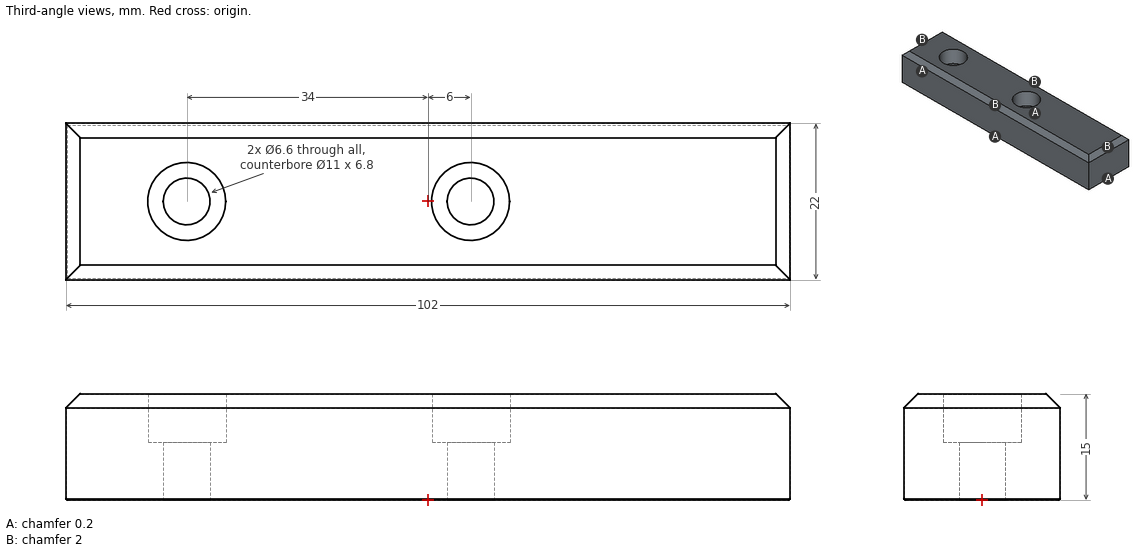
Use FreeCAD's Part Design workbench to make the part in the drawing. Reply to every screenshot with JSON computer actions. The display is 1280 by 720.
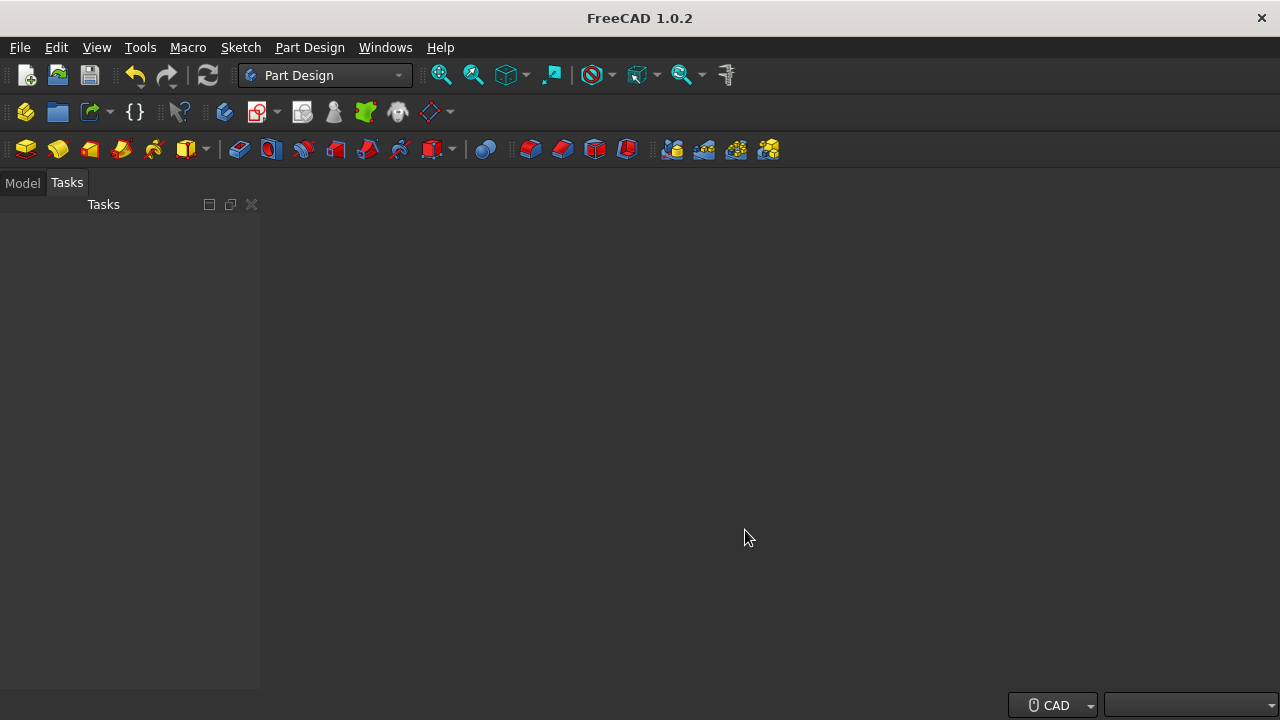
{"action": "left_click", "coordinate": [26, 76]}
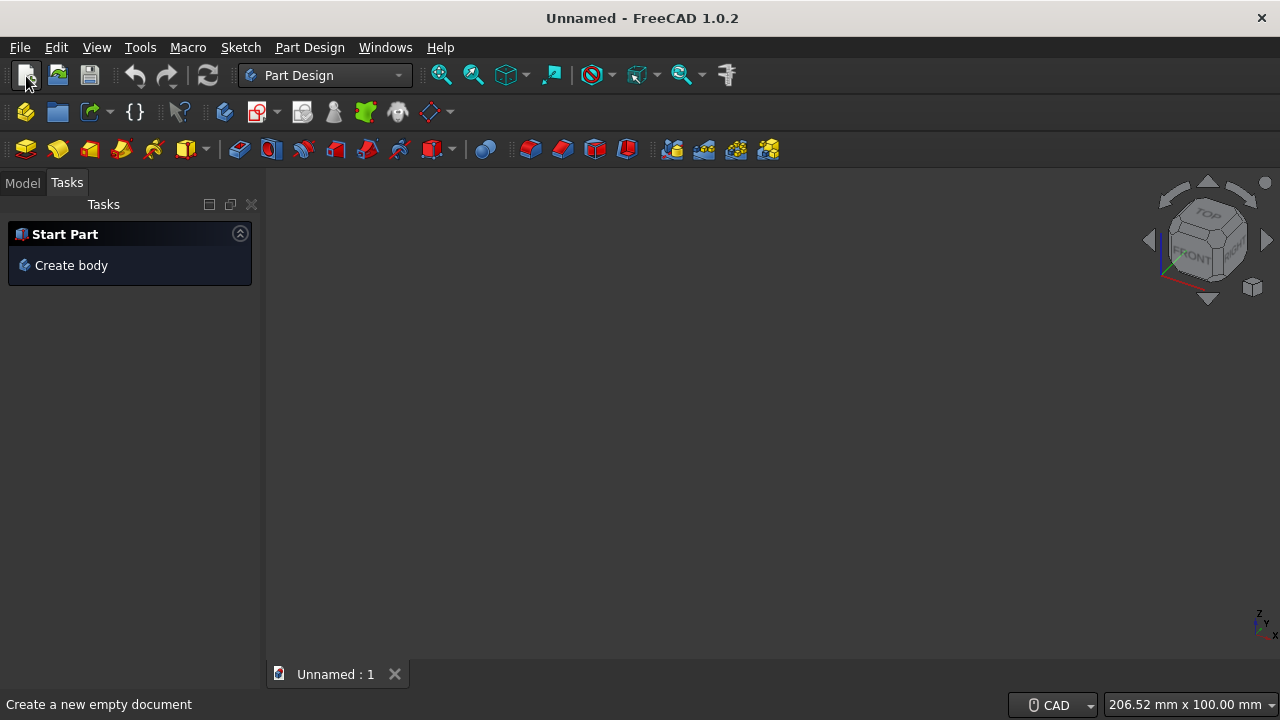
{"action": "left_click", "coordinate": [258, 112]}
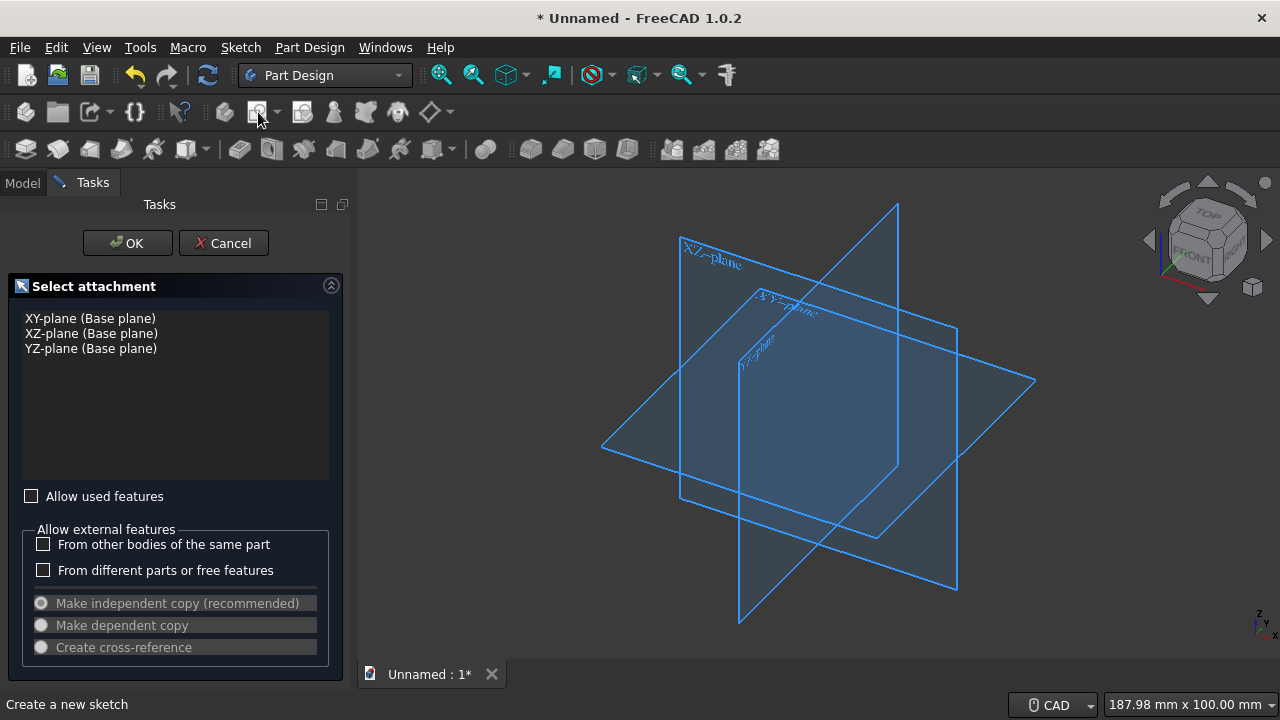
{"action": "left_click", "coordinate": [82, 318]}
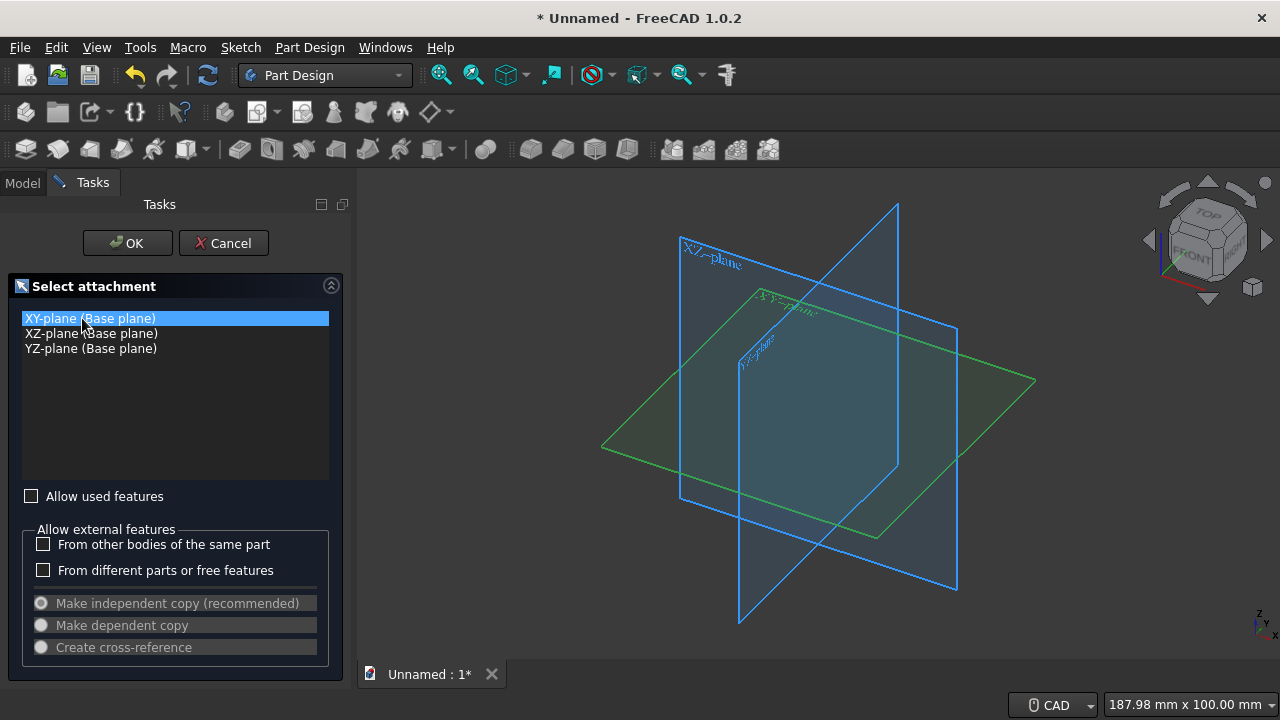
{"action": "left_click", "coordinate": [128, 243]}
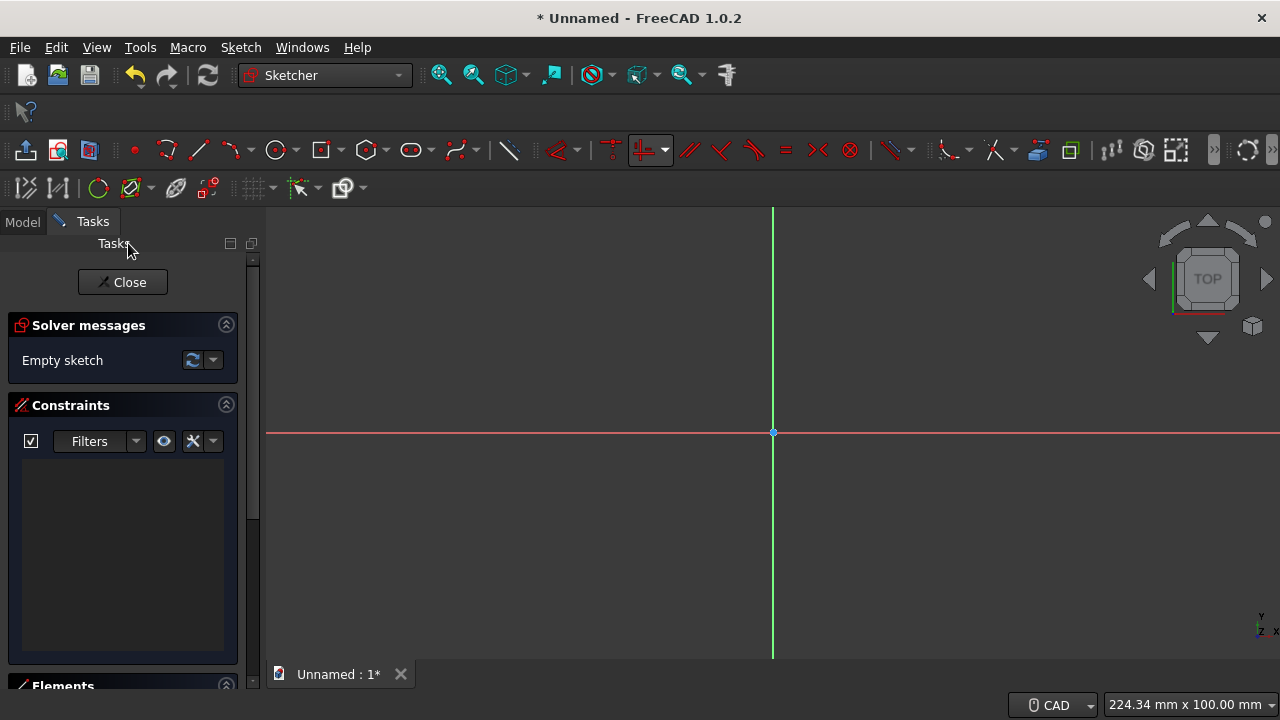
{"action": "left_click", "coordinate": [322, 150]}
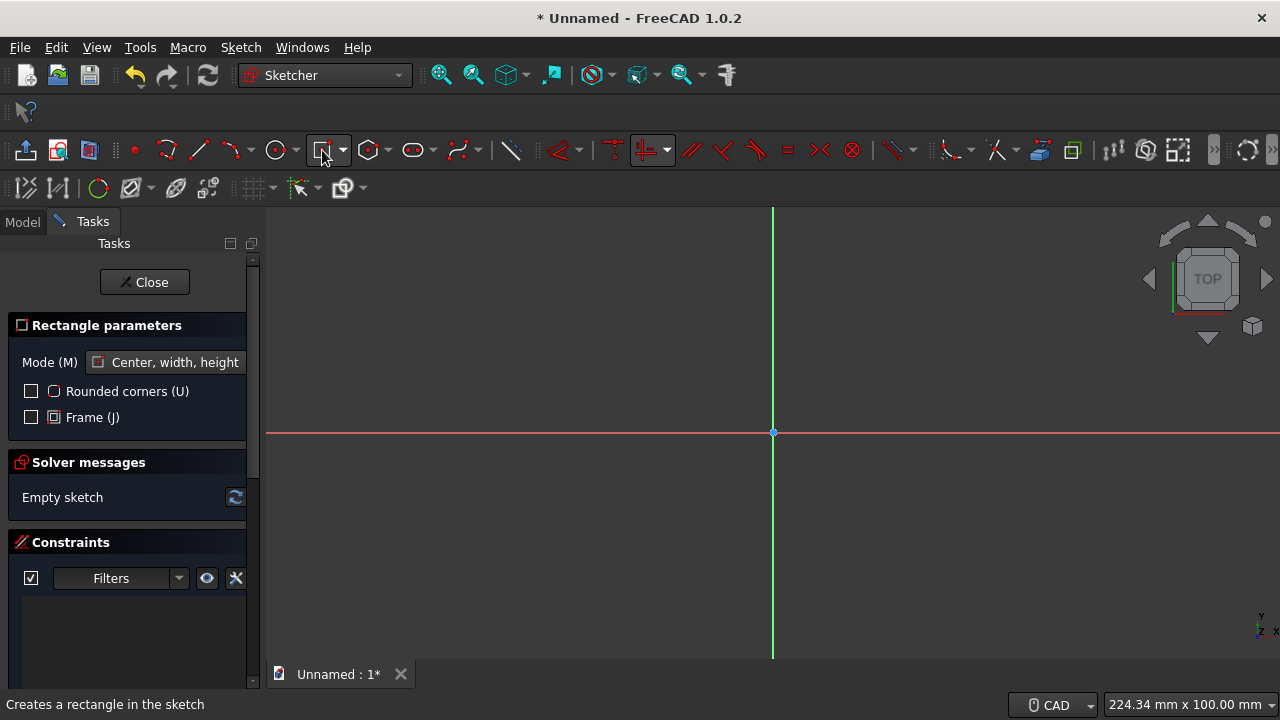
{"action": "left_click", "coordinate": [773, 433]}
{"action": "mouse_move", "coordinate": [1004, 383]}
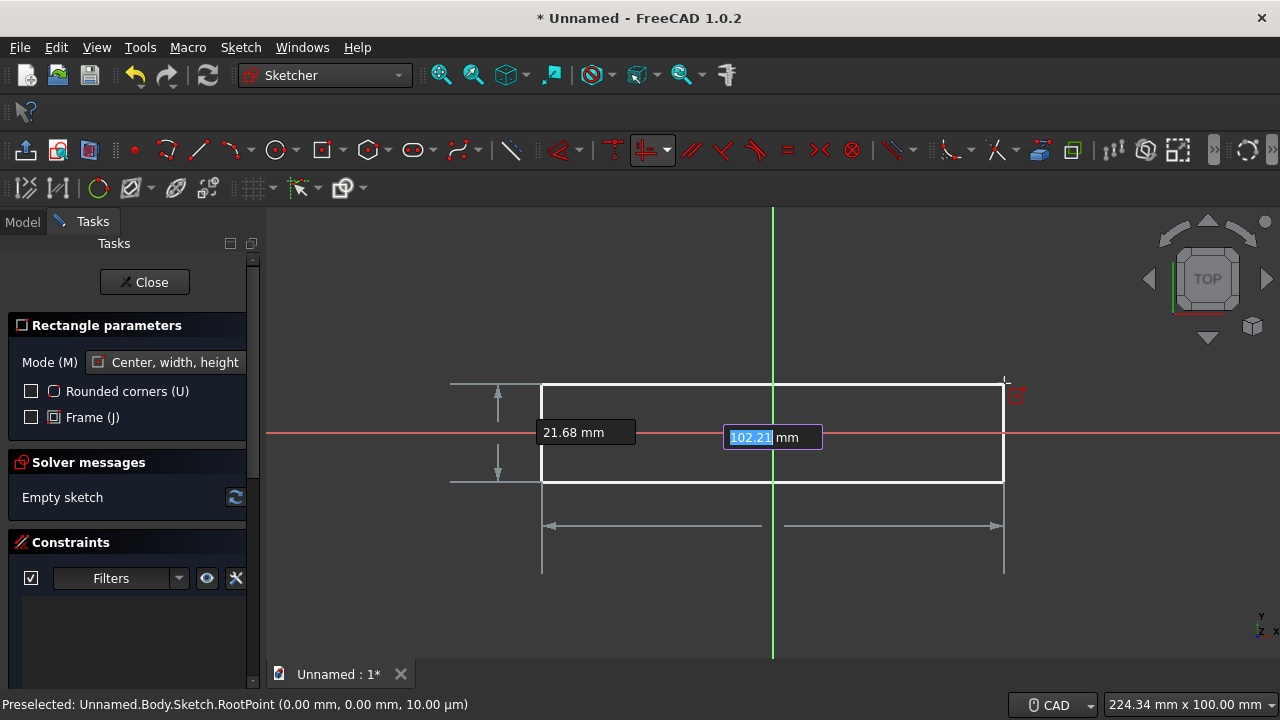
{"action": "type", "text": "102"}
{"action": "key", "text": "Tab"}
{"action": "type", "text": "22"}
{"action": "key", "text": "Return"}
{"action": "key", "text": "Escape"}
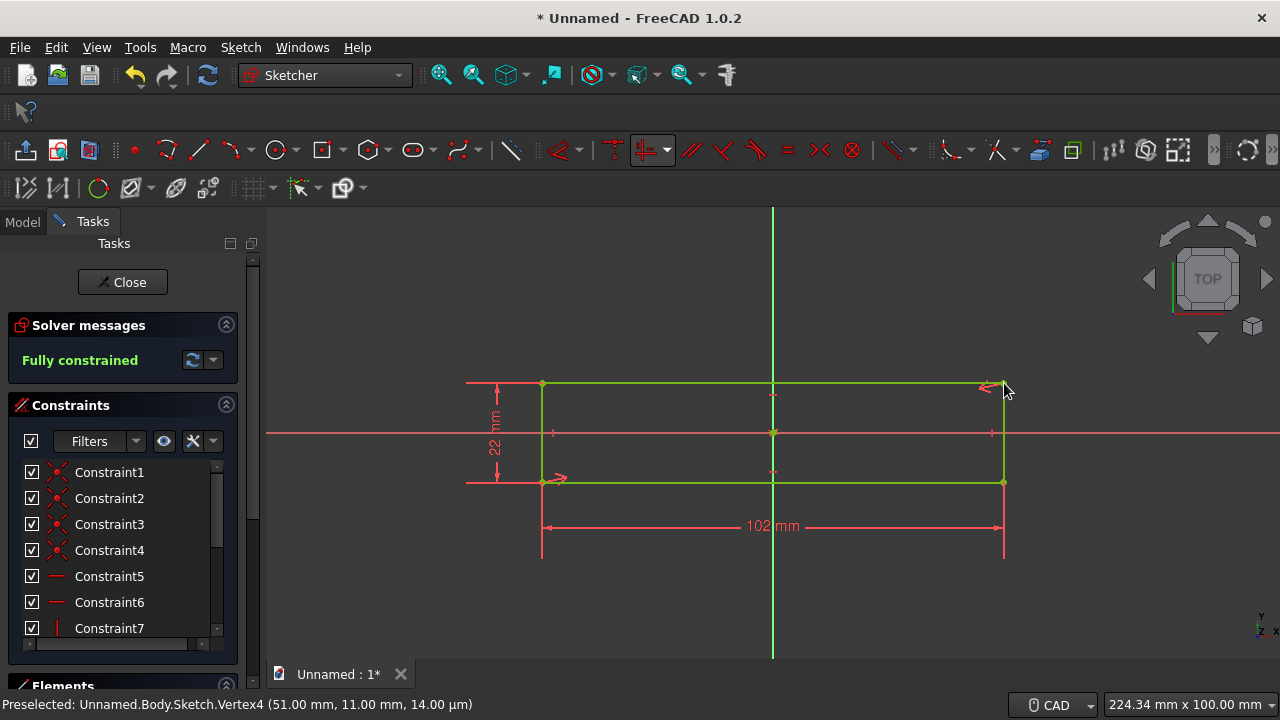
{"action": "left_click", "coordinate": [123, 282]}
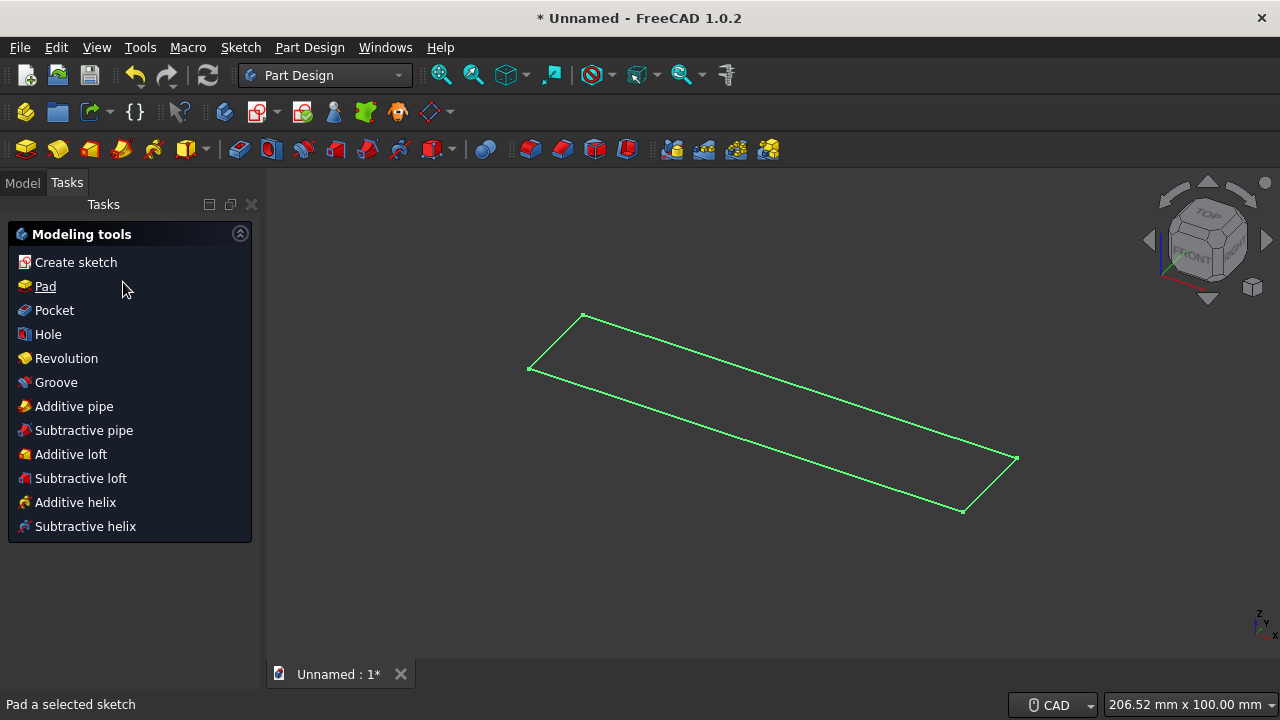
{"action": "left_click", "coordinate": [26, 150]}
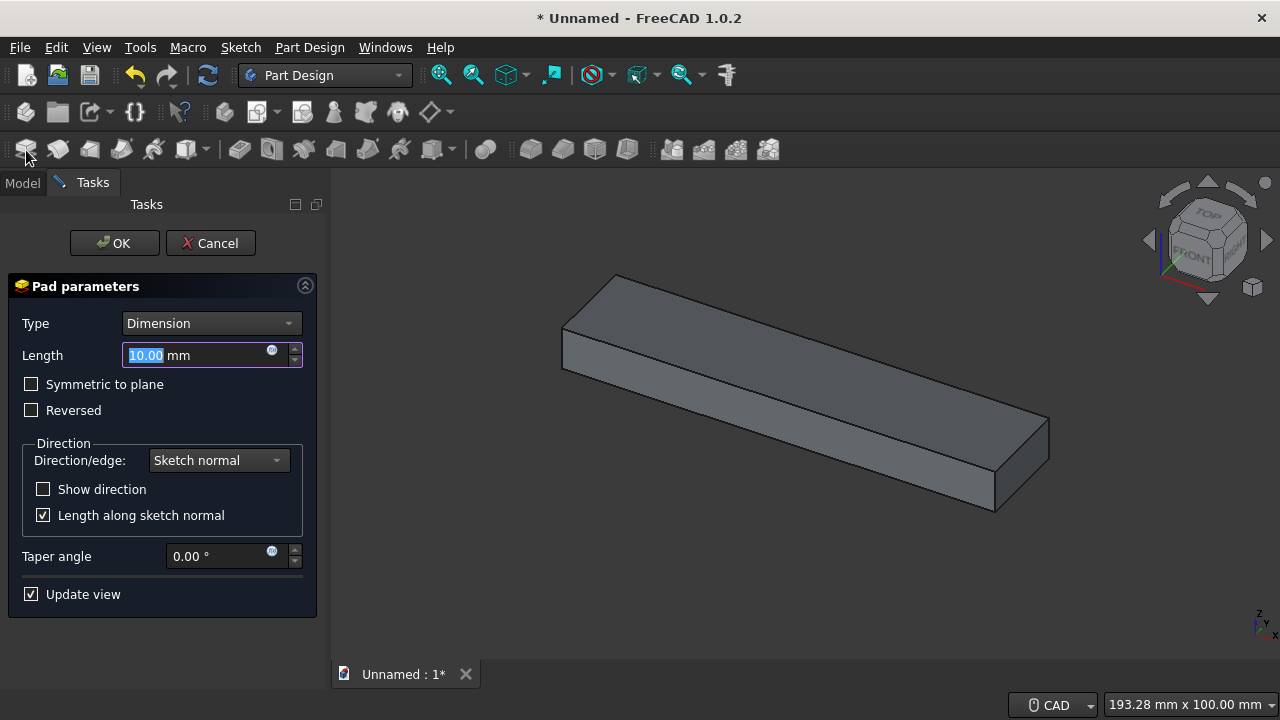
{"action": "type", "text": "15"}
{"action": "key", "text": "Tab"}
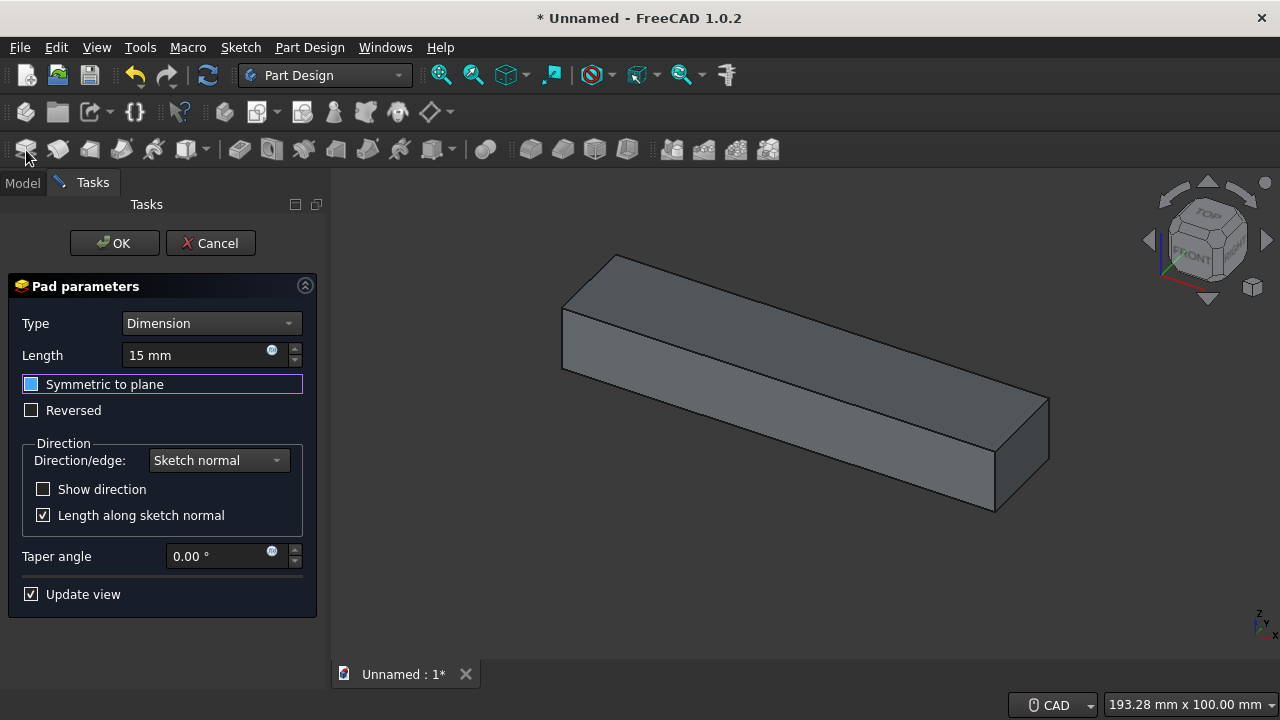
{"action": "left_click", "coordinate": [115, 243]}